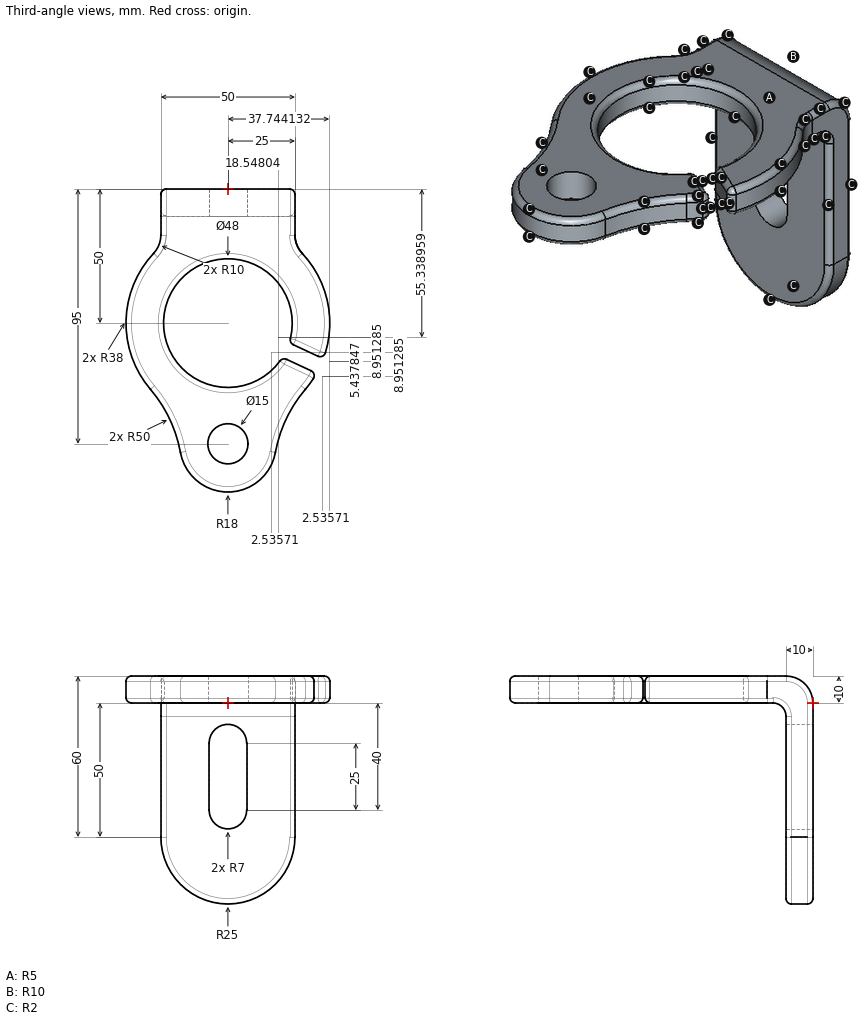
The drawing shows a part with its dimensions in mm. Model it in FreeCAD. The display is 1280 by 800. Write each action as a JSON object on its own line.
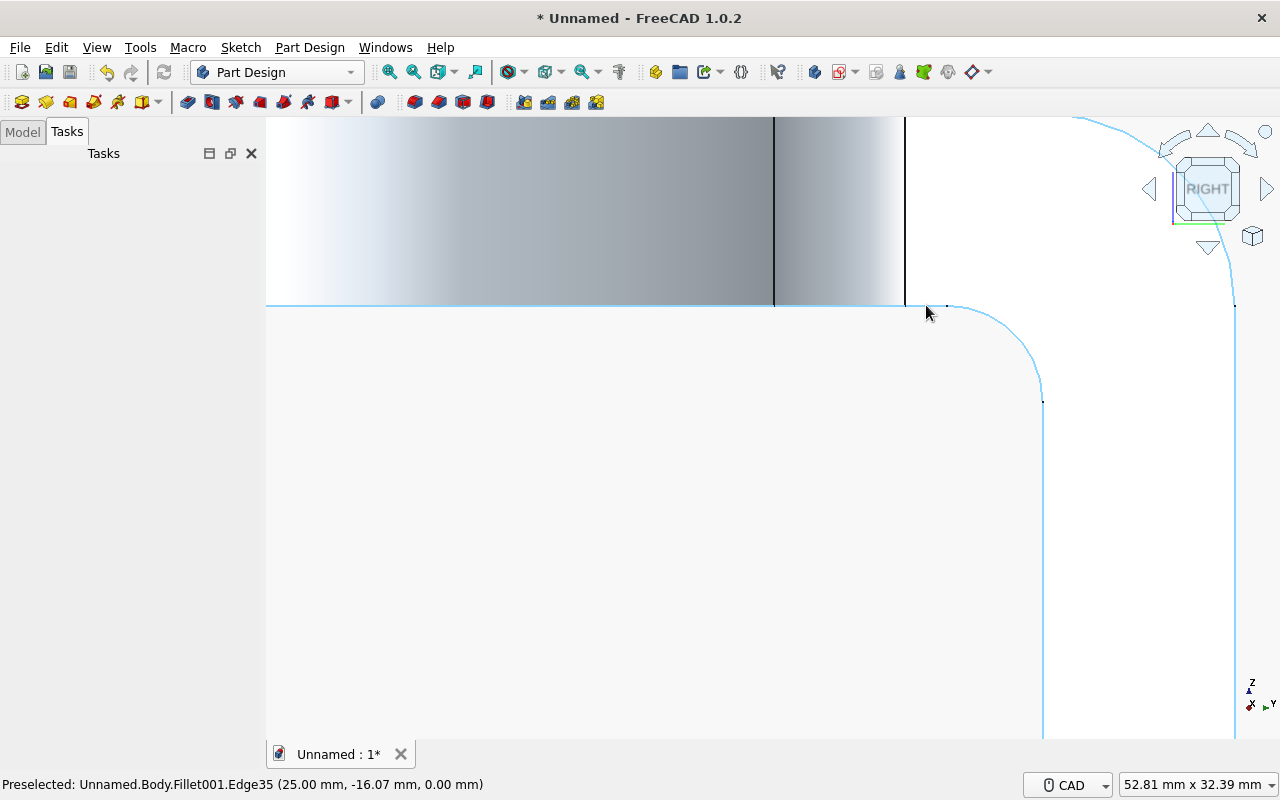
{"action": "left_click", "coordinate": [390, 72]}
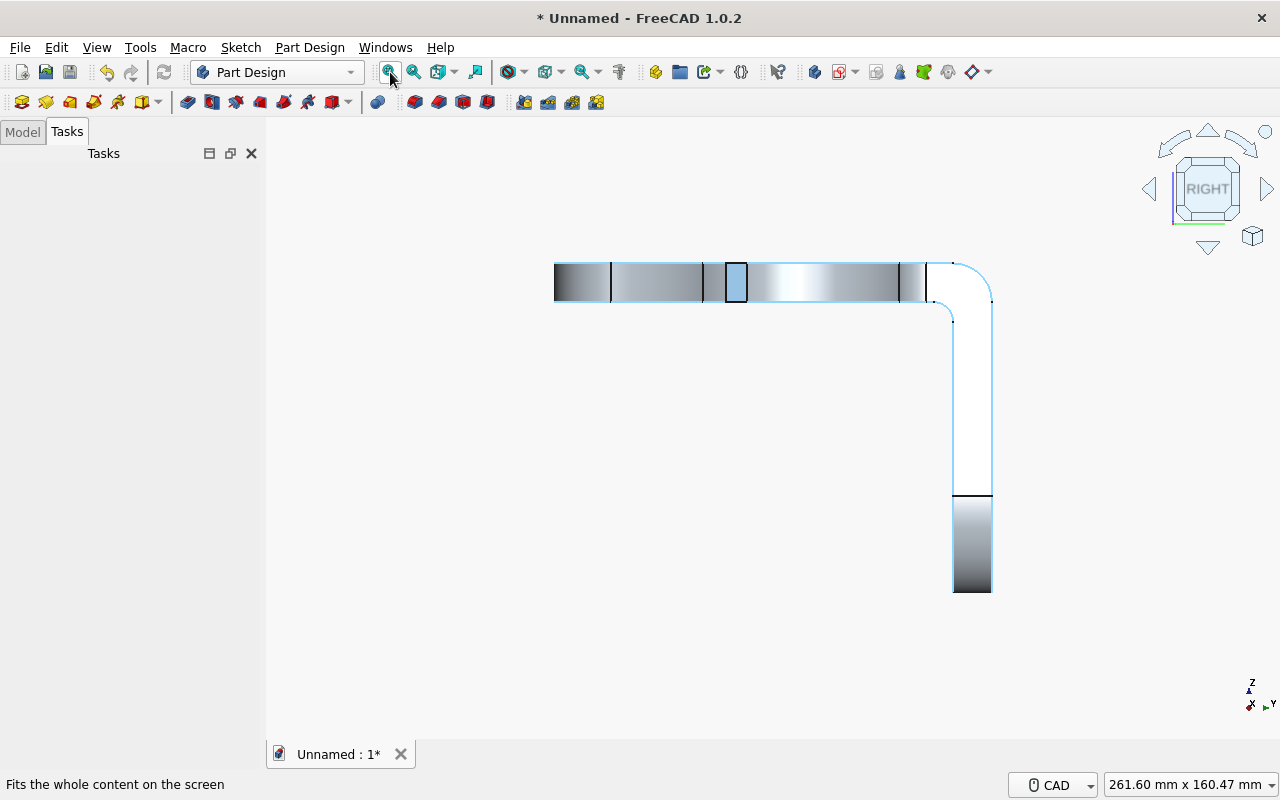
{"action": "key", "text": "5"}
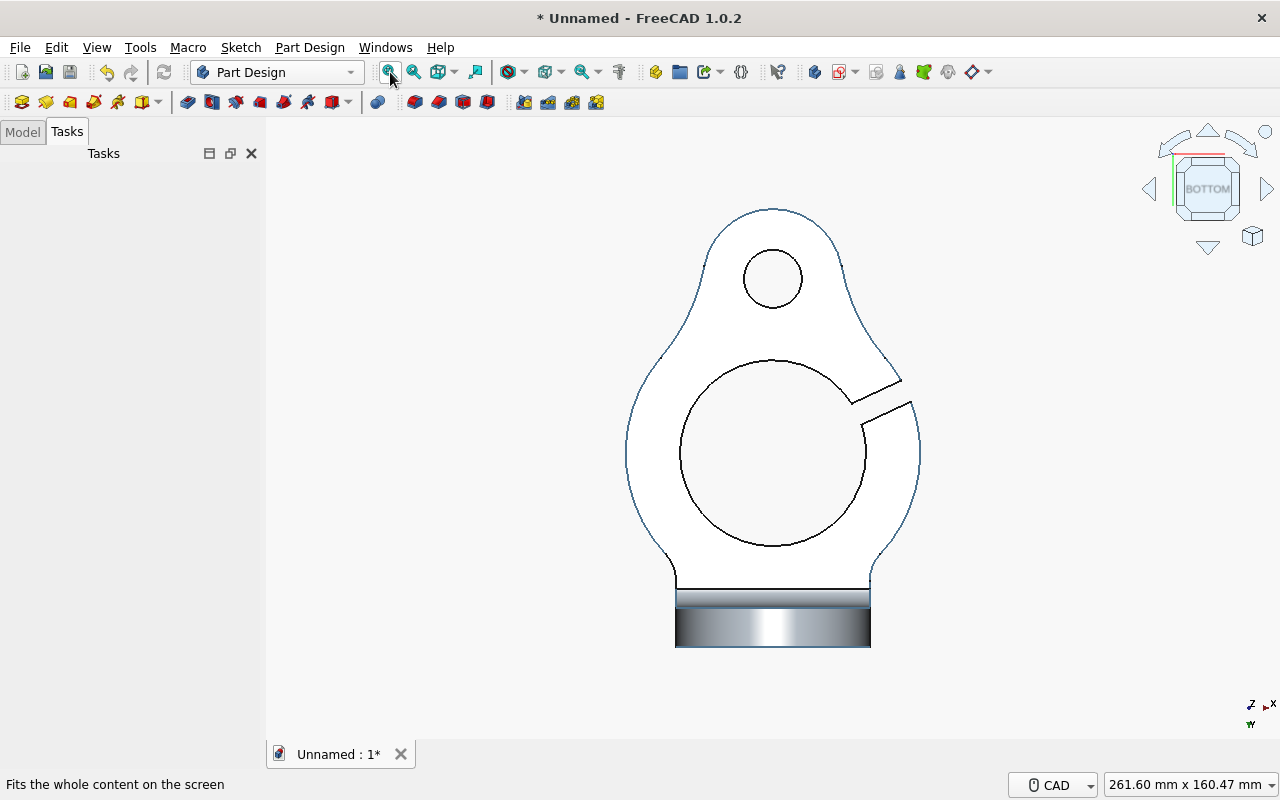
{"action": "left_click", "coordinate": [673, 565], "text": "ctrl"}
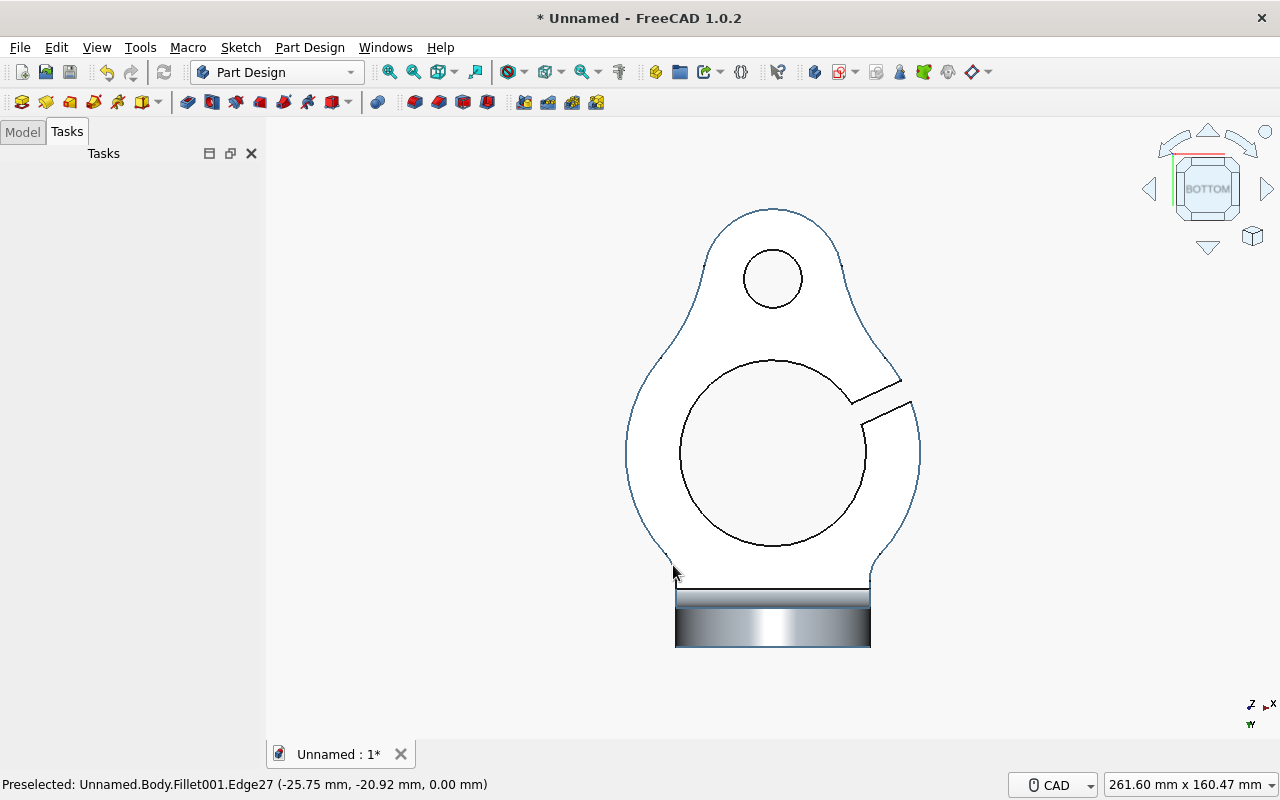
{"action": "left_click", "coordinate": [684, 478], "text": "ctrl"}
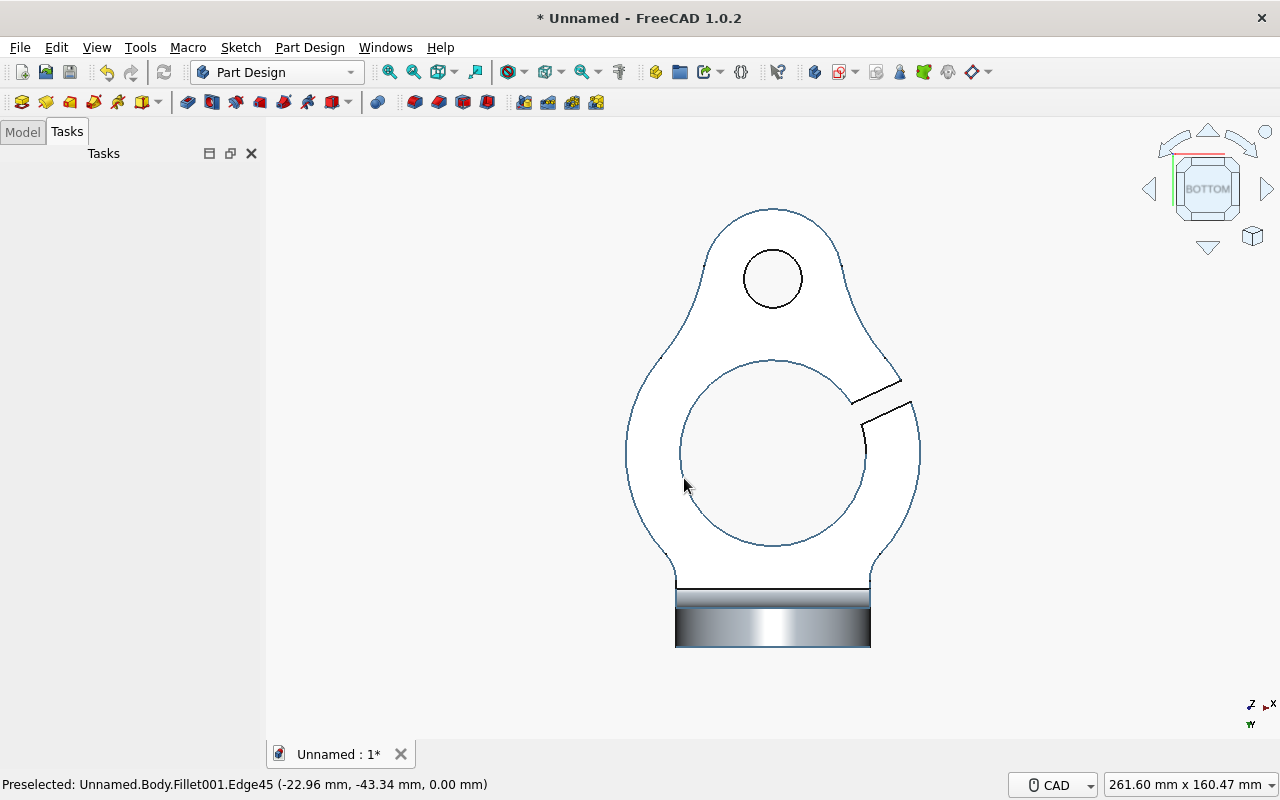
{"action": "scroll", "coordinate": [676, 584], "scroll_direction": "up", "scroll_amount": 8}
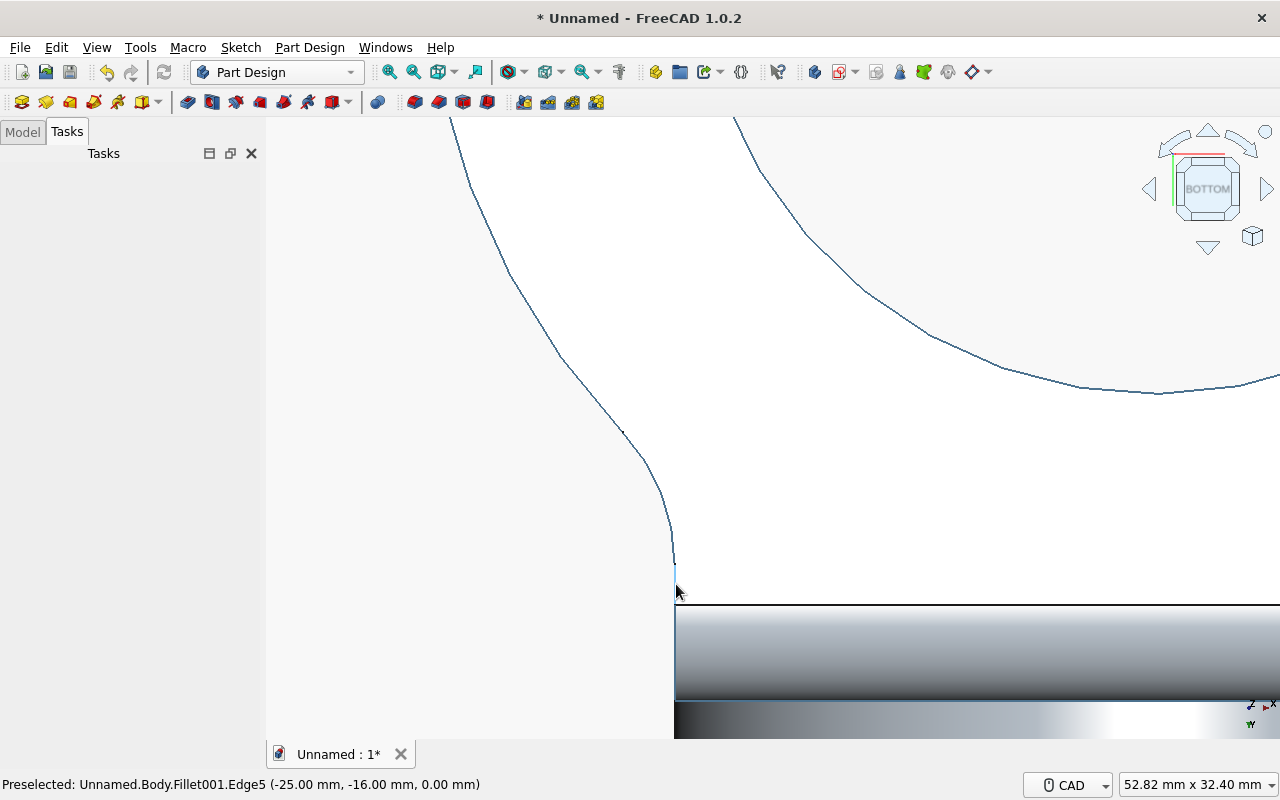
{"action": "left_click", "coordinate": [675, 583], "text": "ctrl"}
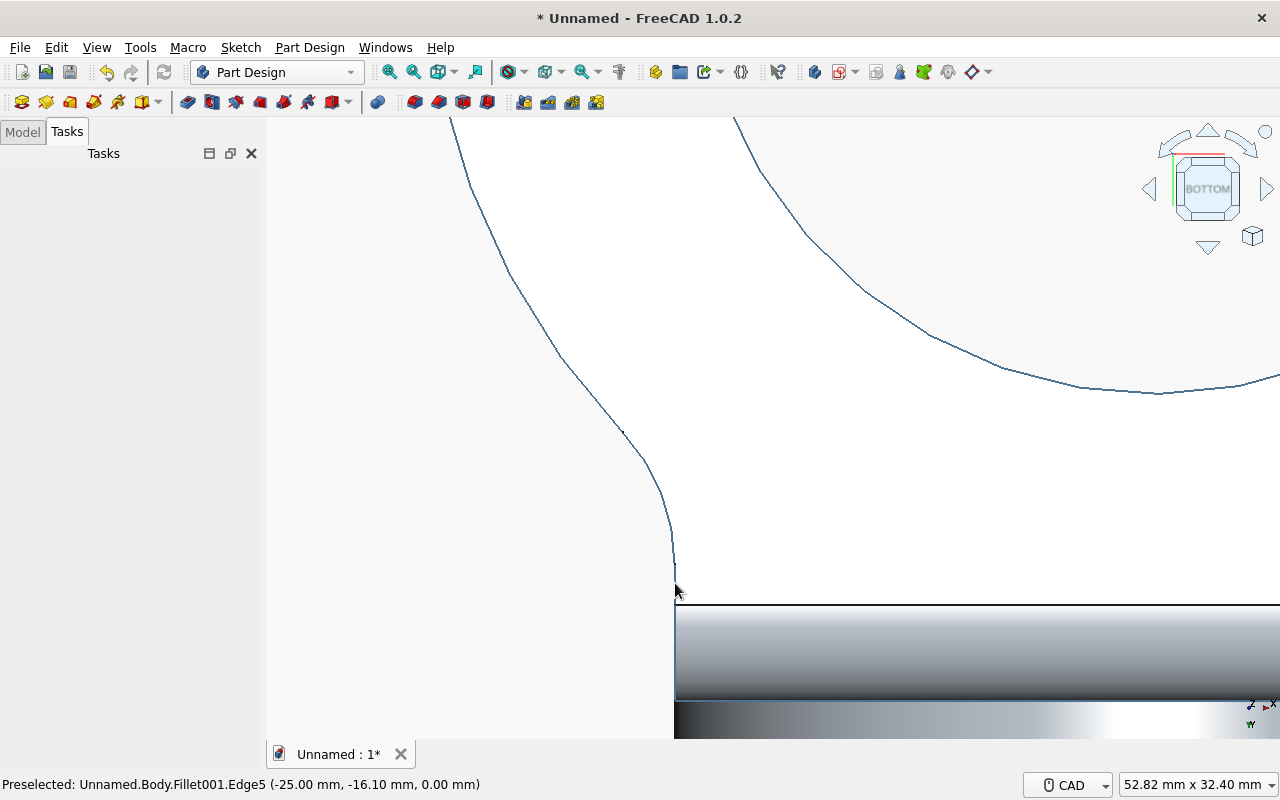
{"action": "left_click", "coordinate": [390, 72]}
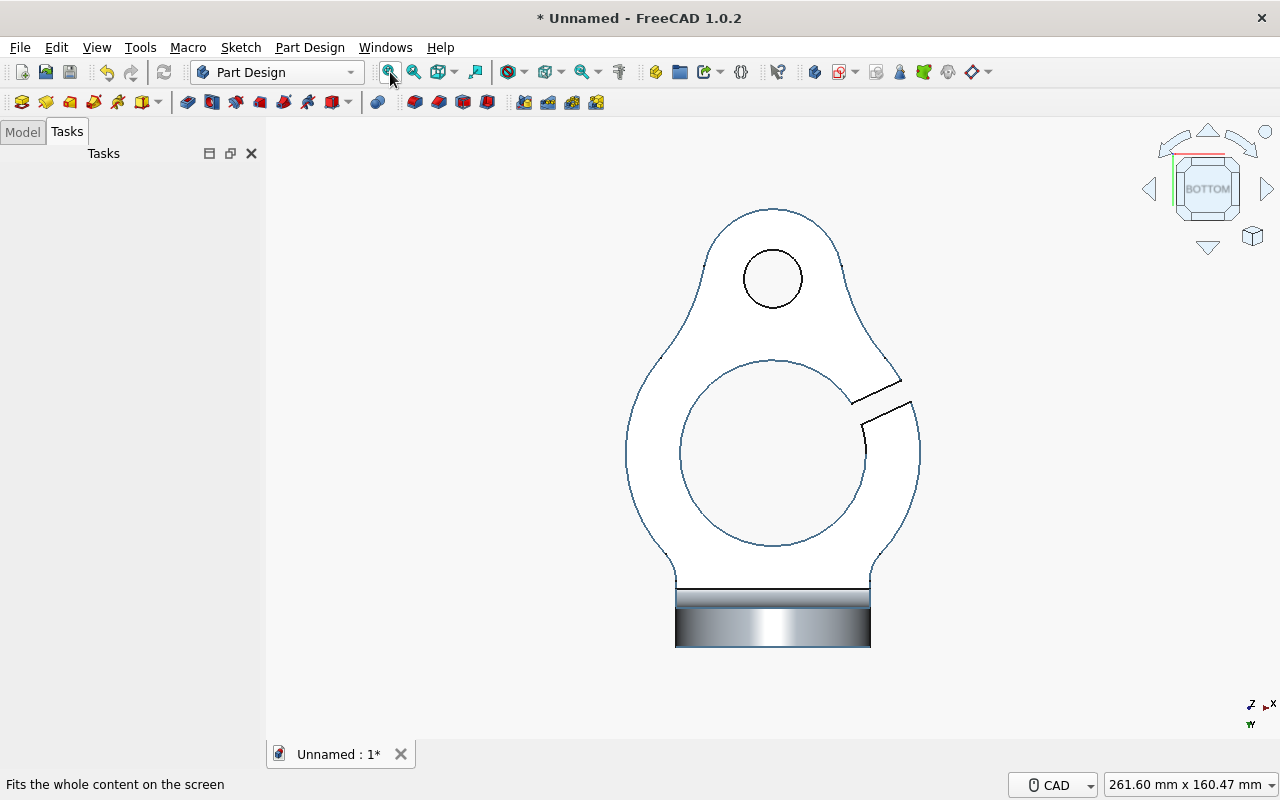
{"action": "key", "text": "4"}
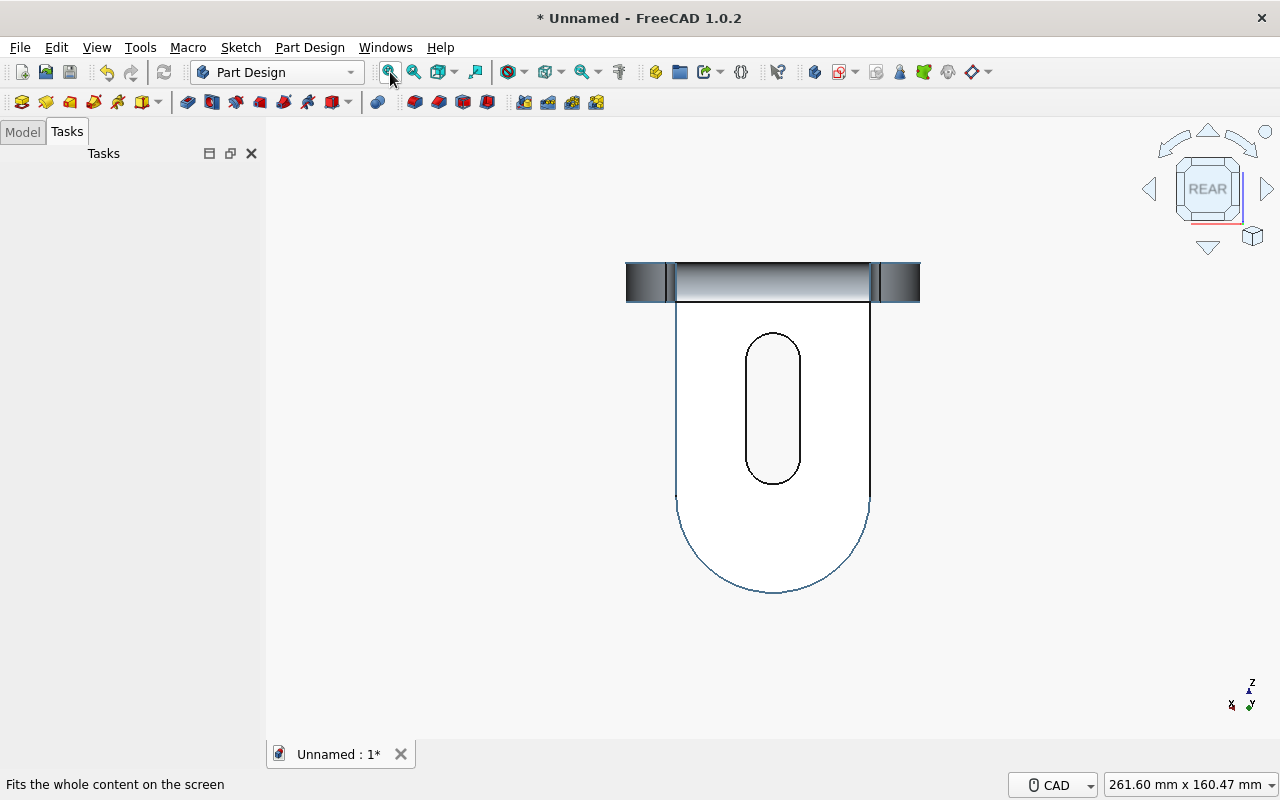
{"action": "key", "text": "6"}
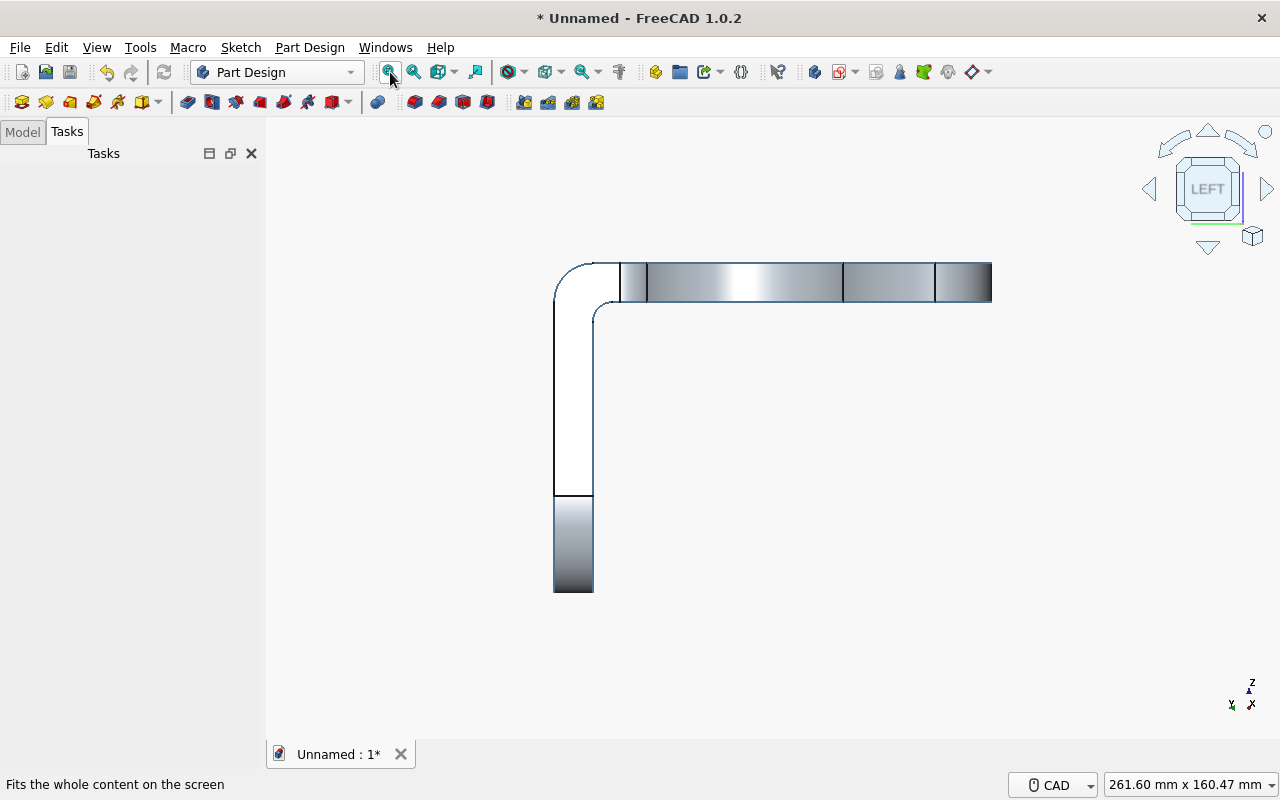
{"action": "left_click", "coordinate": [554, 398], "text": "ctrl"}